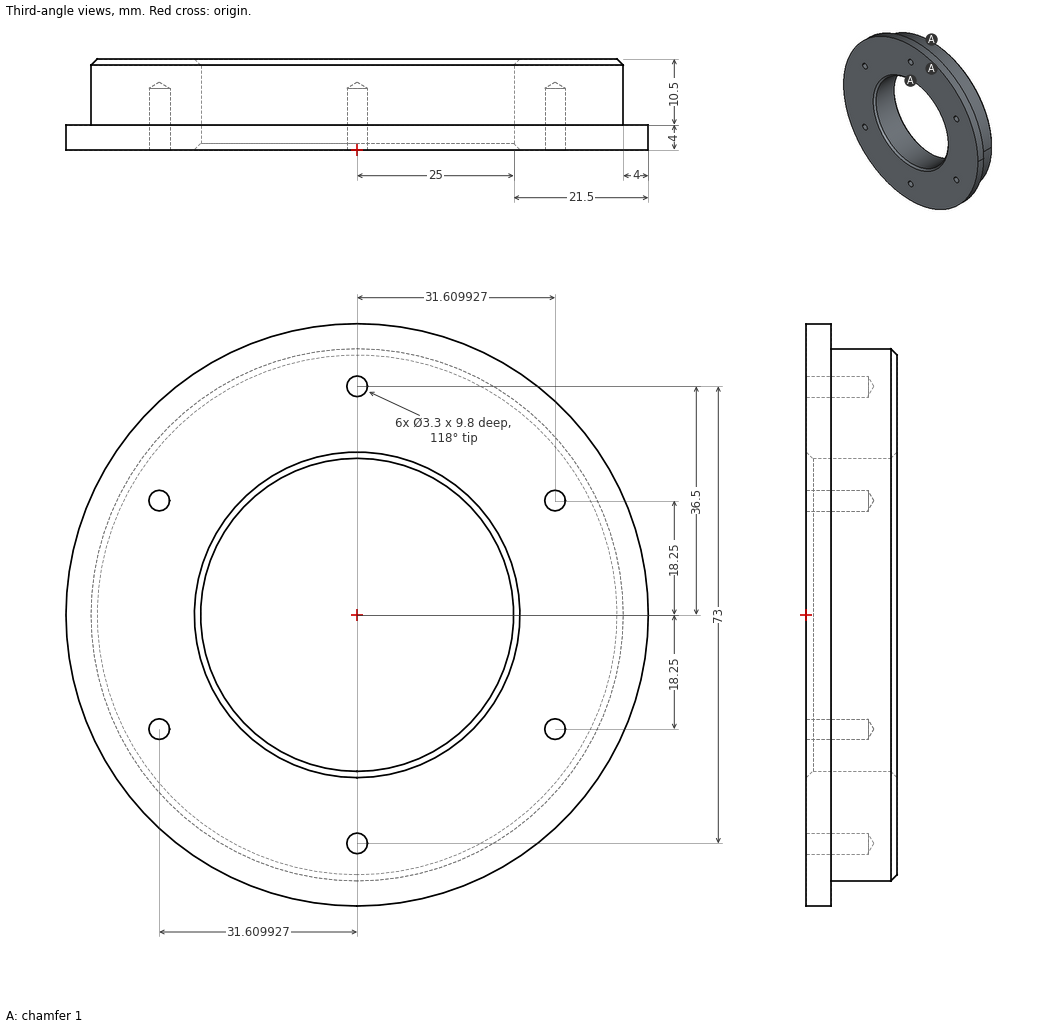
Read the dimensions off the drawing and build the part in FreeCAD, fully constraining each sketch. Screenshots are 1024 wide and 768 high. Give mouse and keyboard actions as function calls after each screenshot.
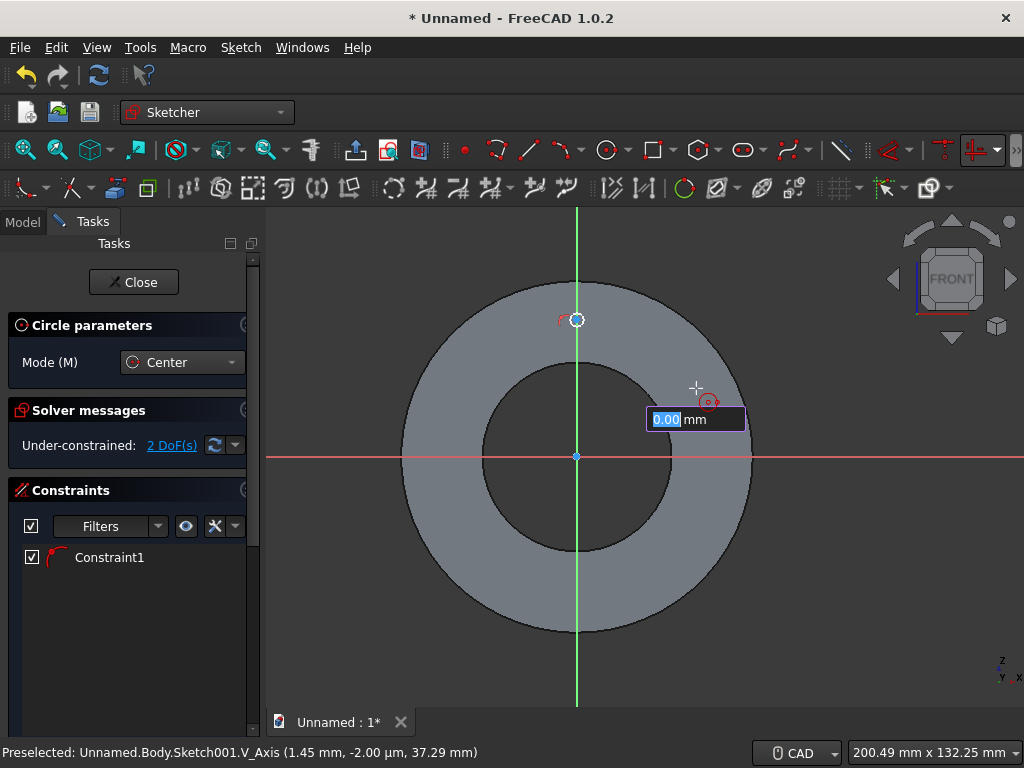
scroll(701, 384, up, 5)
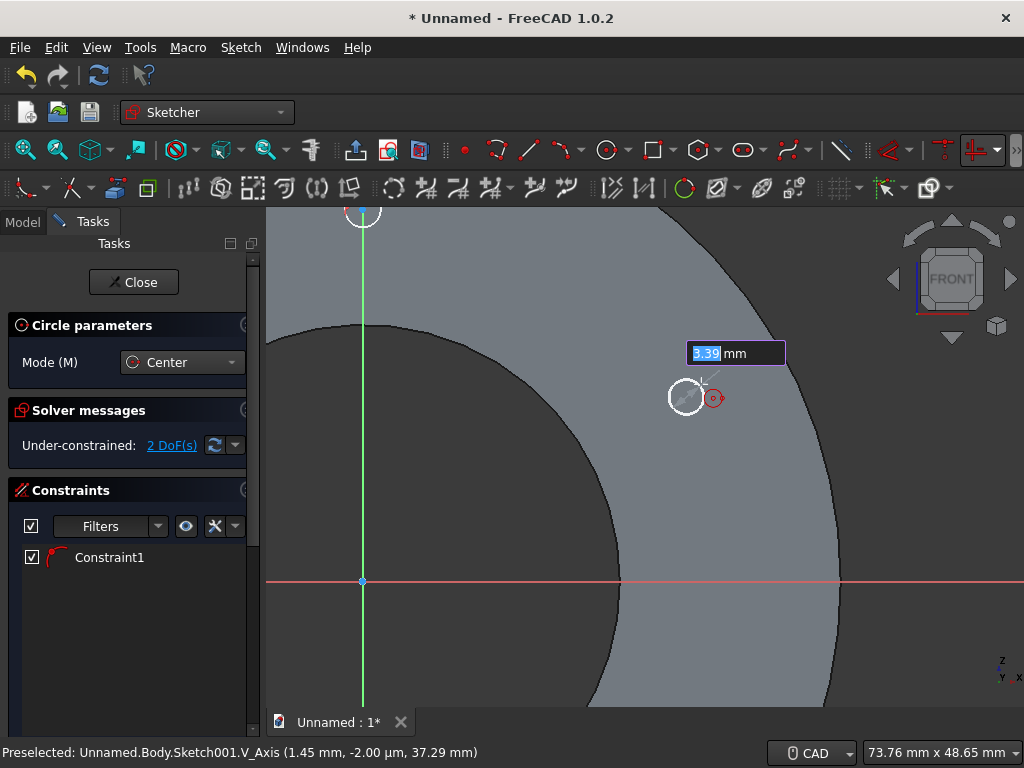
click(700, 382)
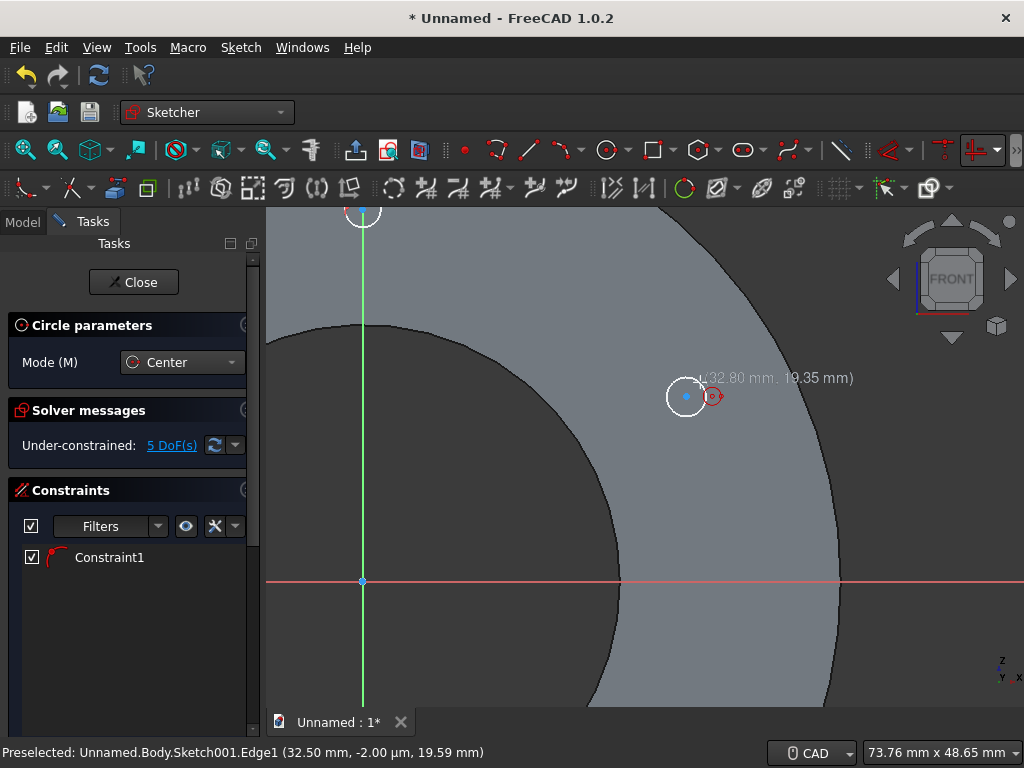
scroll(701, 384, down, 5)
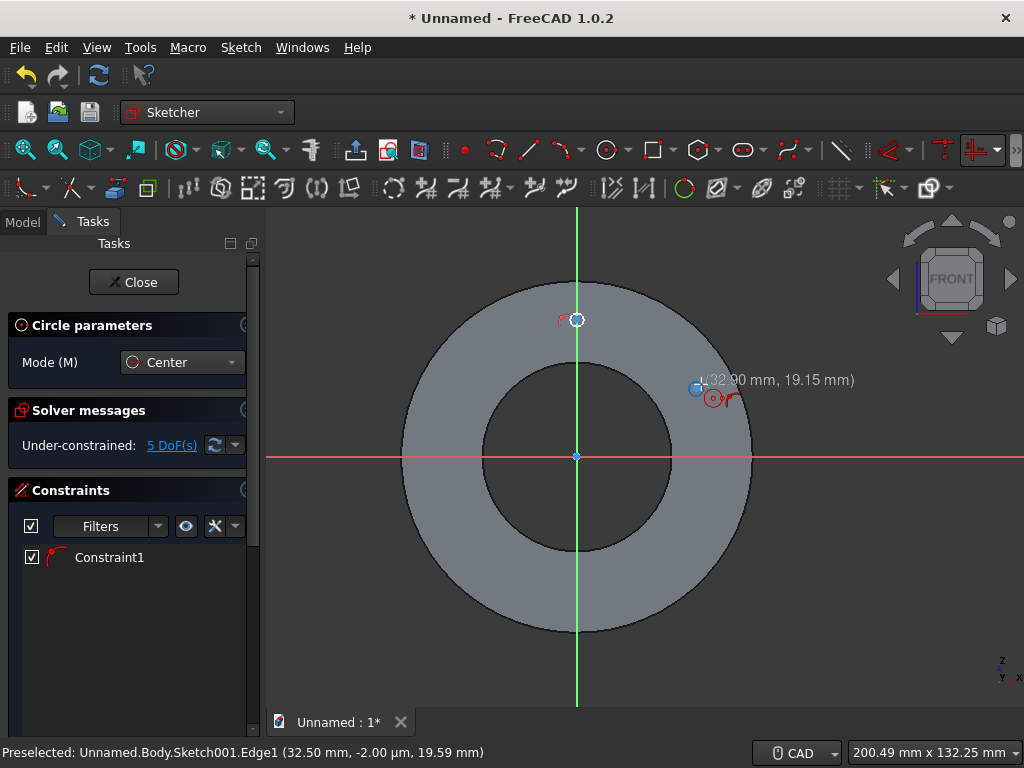
scroll(696, 526, up, 7)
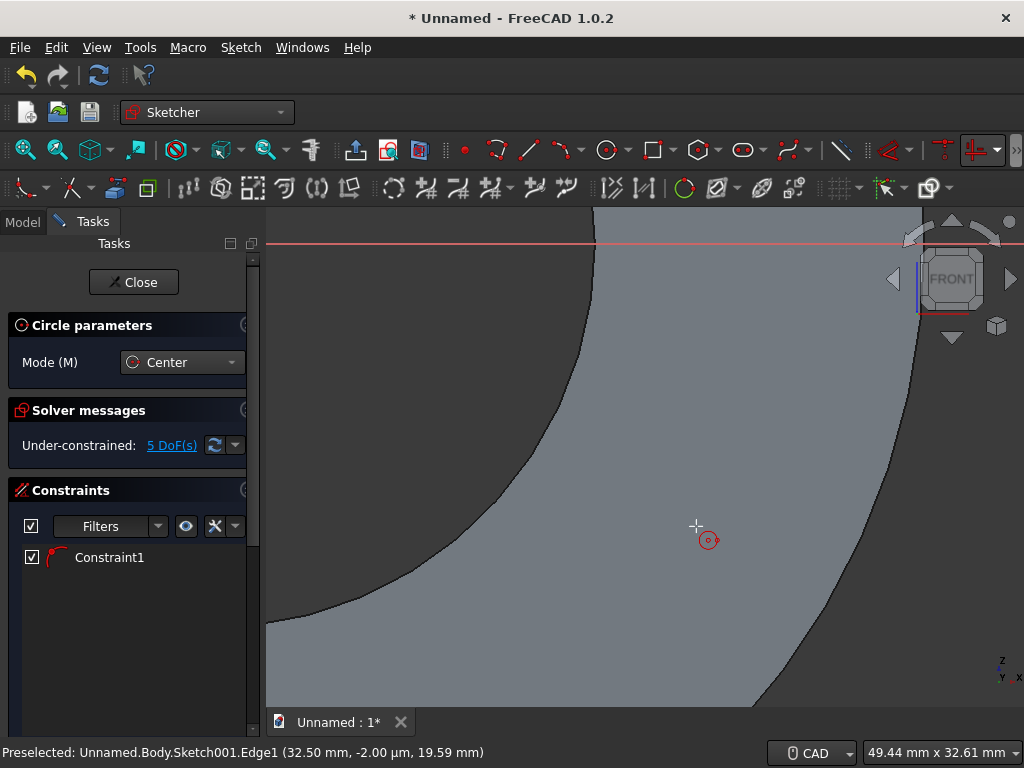
scroll(696, 527, down, 7)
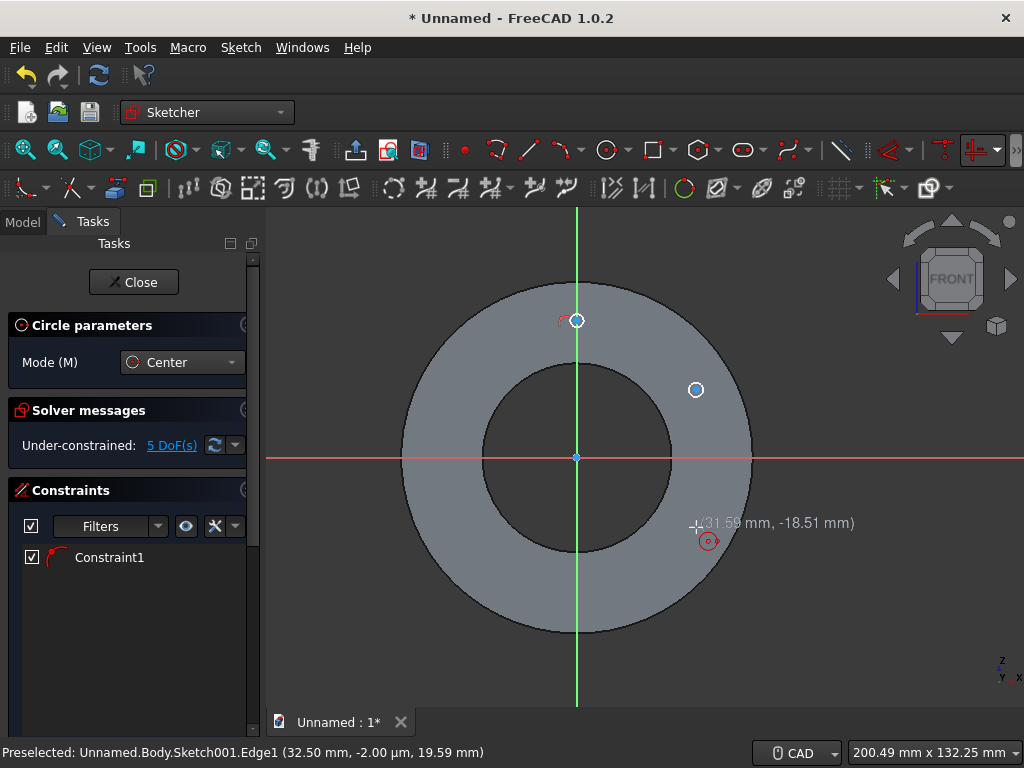
click(696, 527)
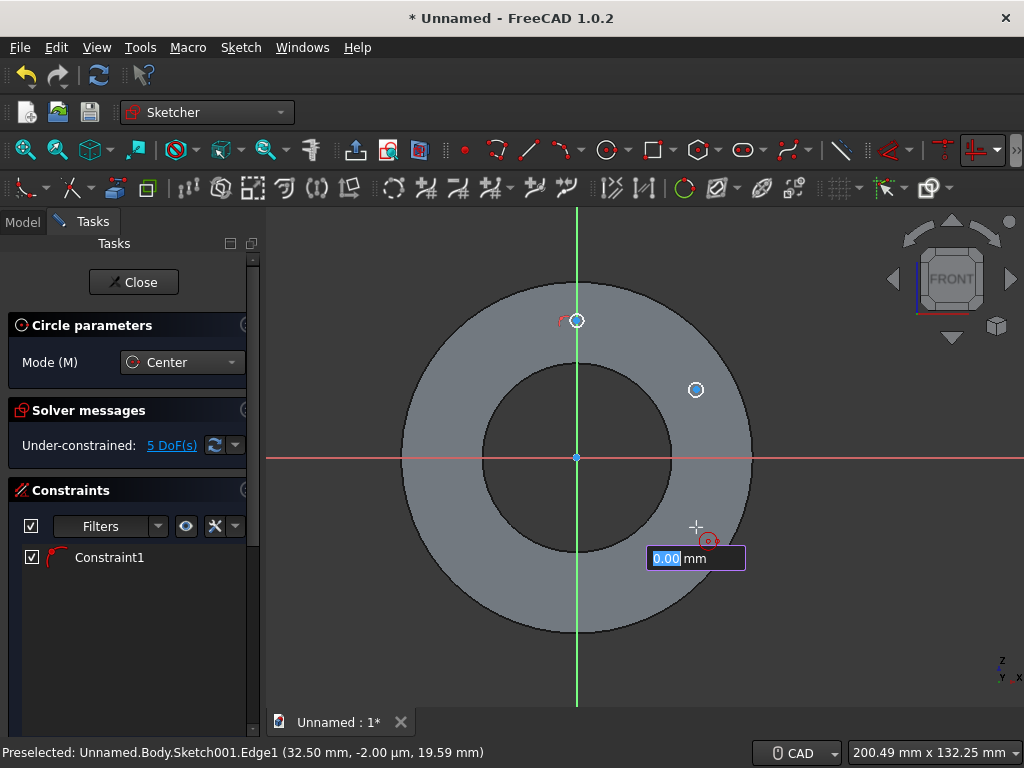
scroll(701, 522, up, 5)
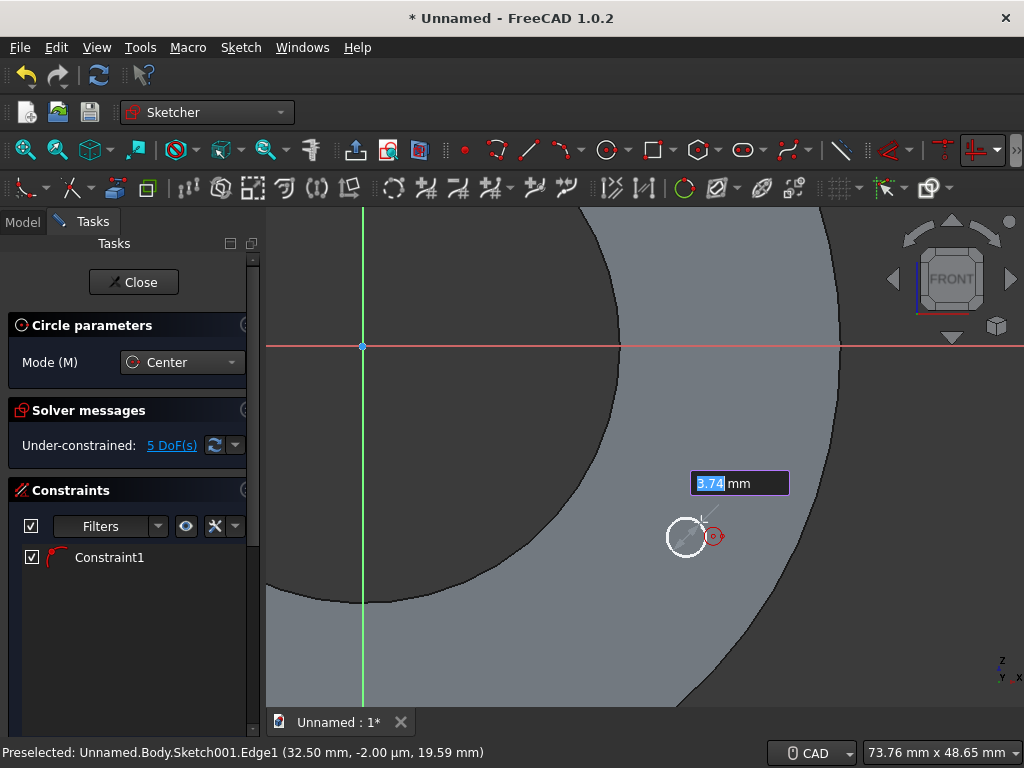
click(700, 522)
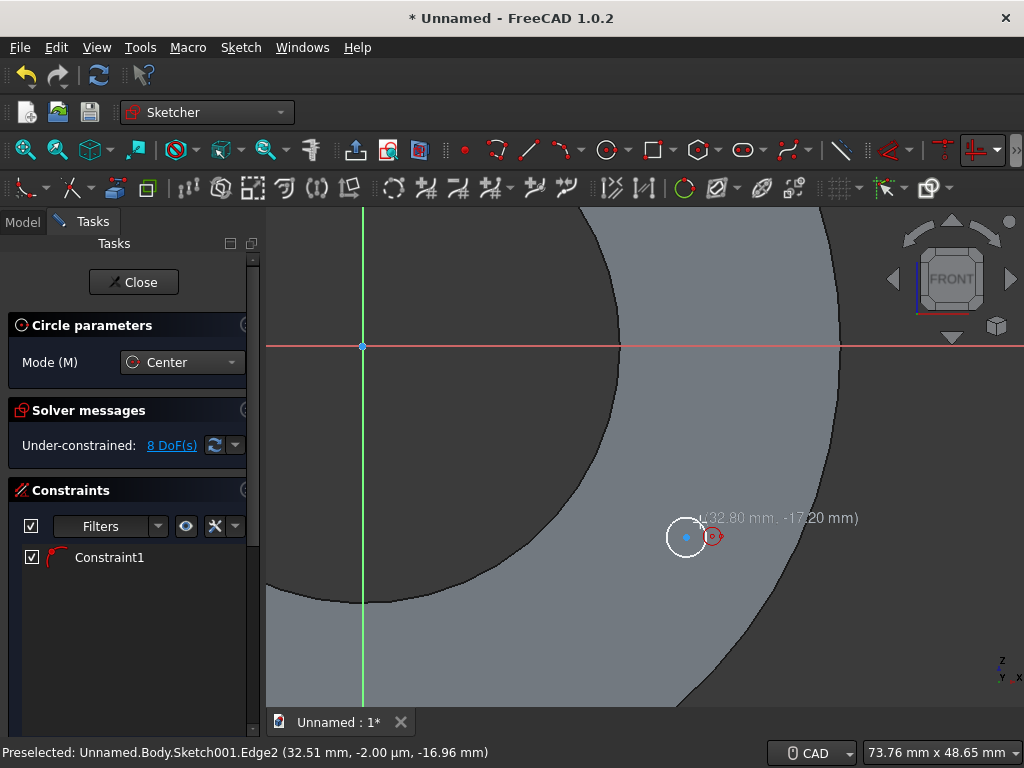
scroll(701, 521, down, 5)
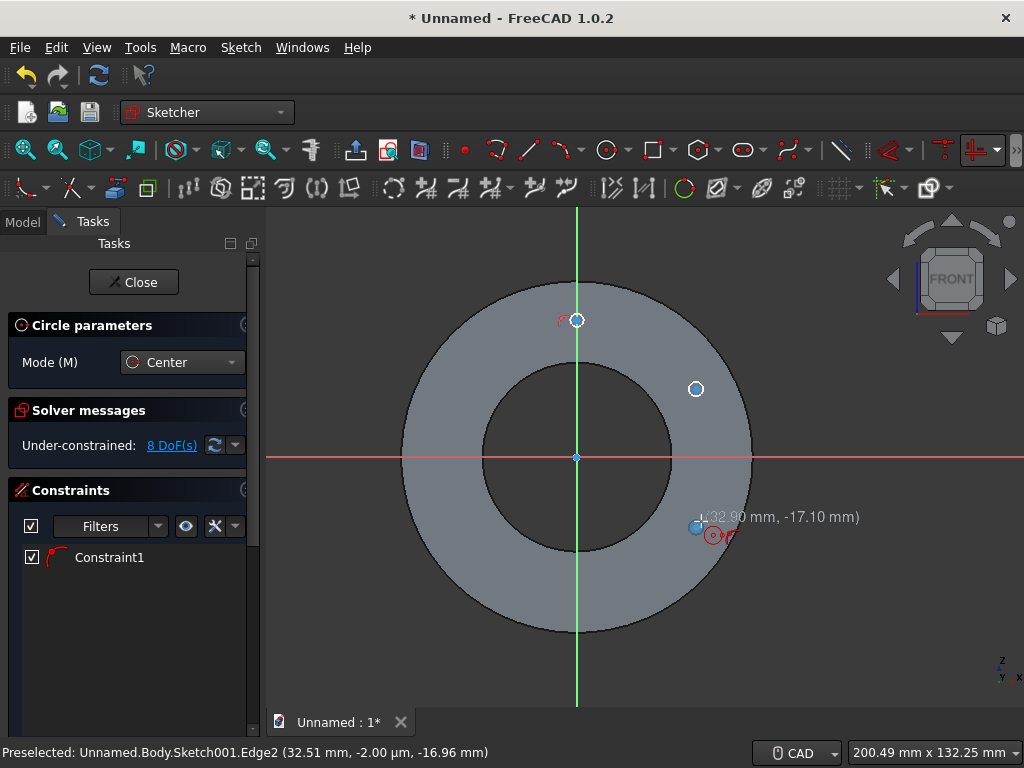
scroll(577, 595, up, 7)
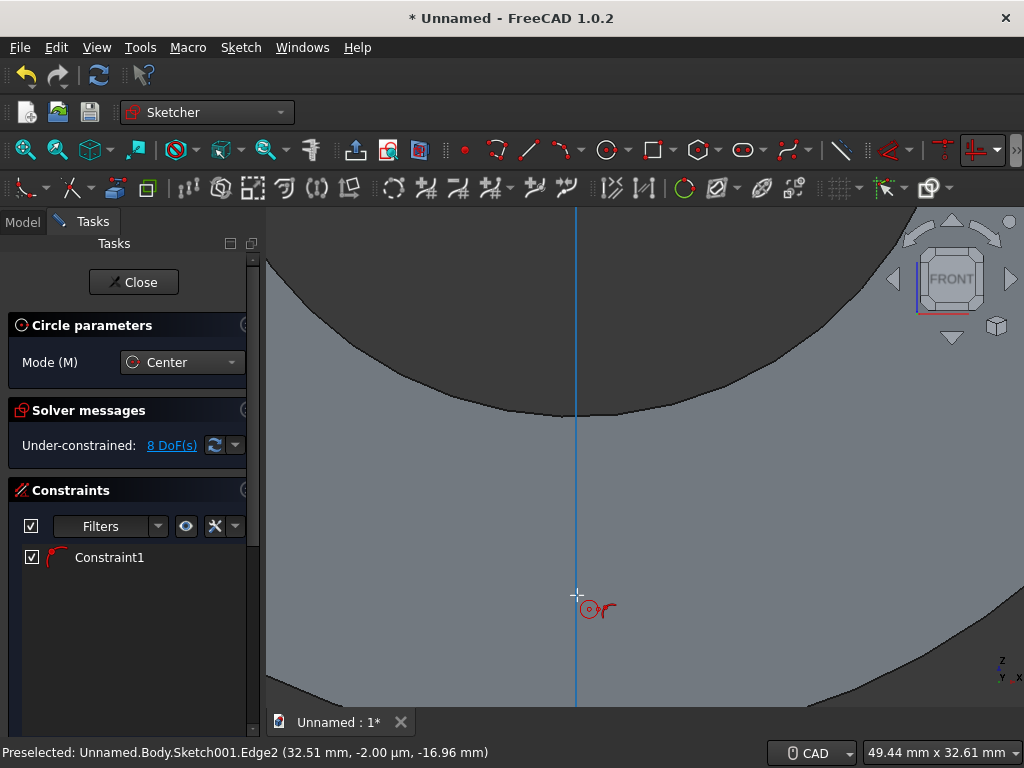
scroll(577, 596, down, 7)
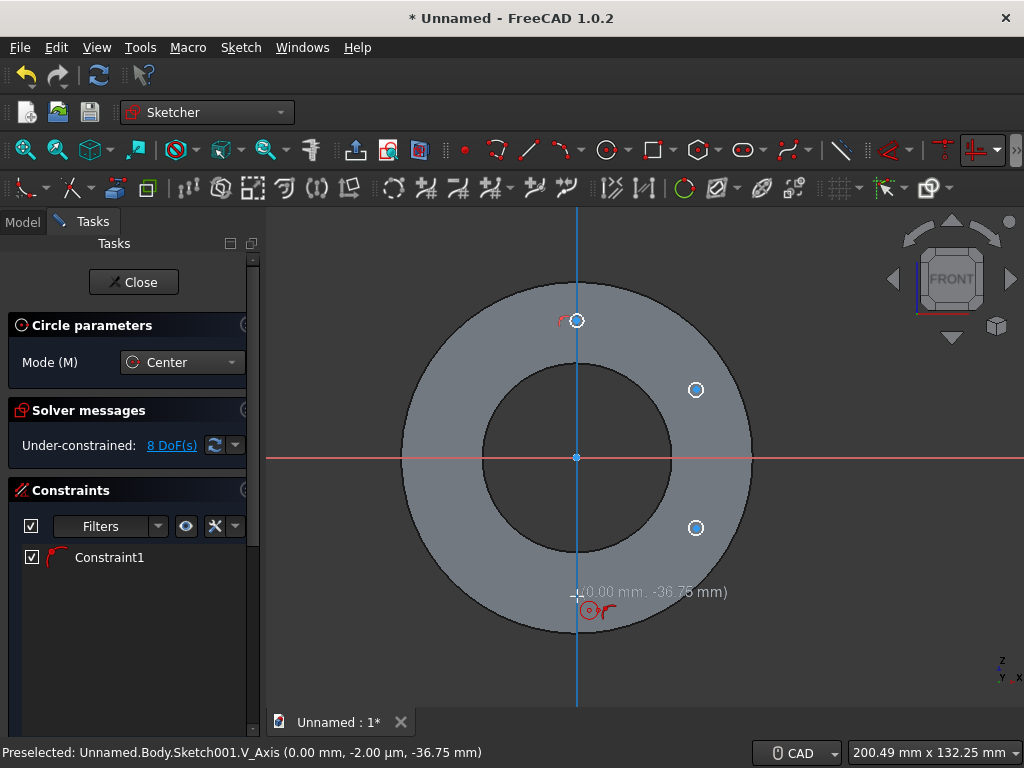
click(577, 596)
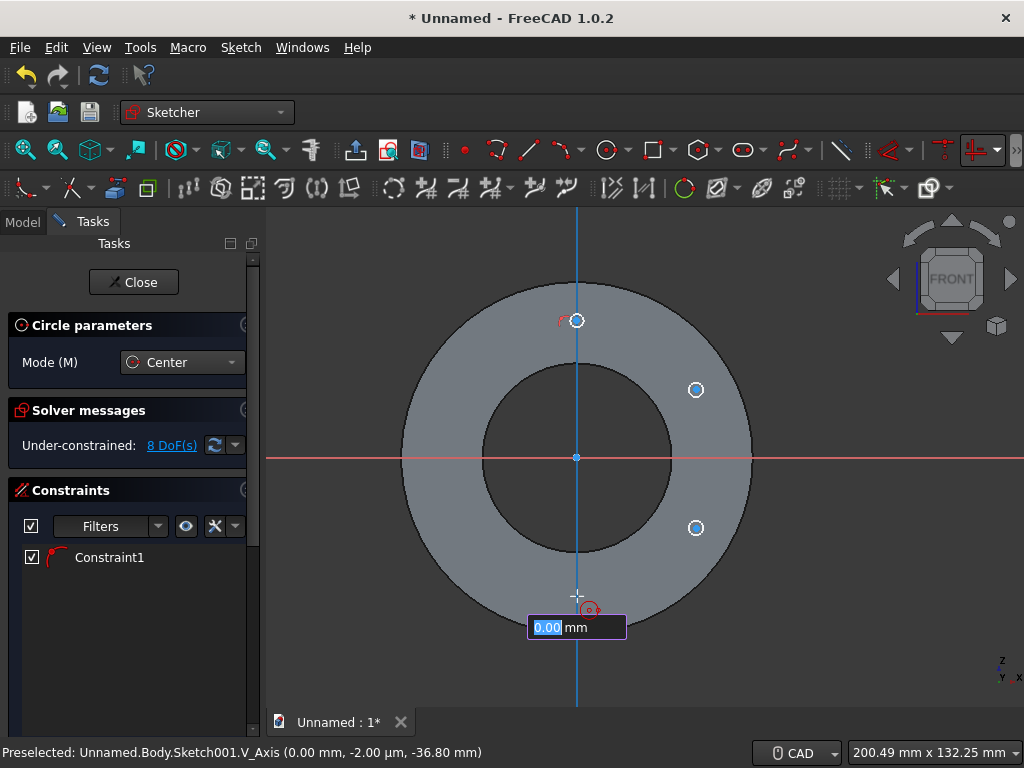
scroll(583, 594, up, 5)